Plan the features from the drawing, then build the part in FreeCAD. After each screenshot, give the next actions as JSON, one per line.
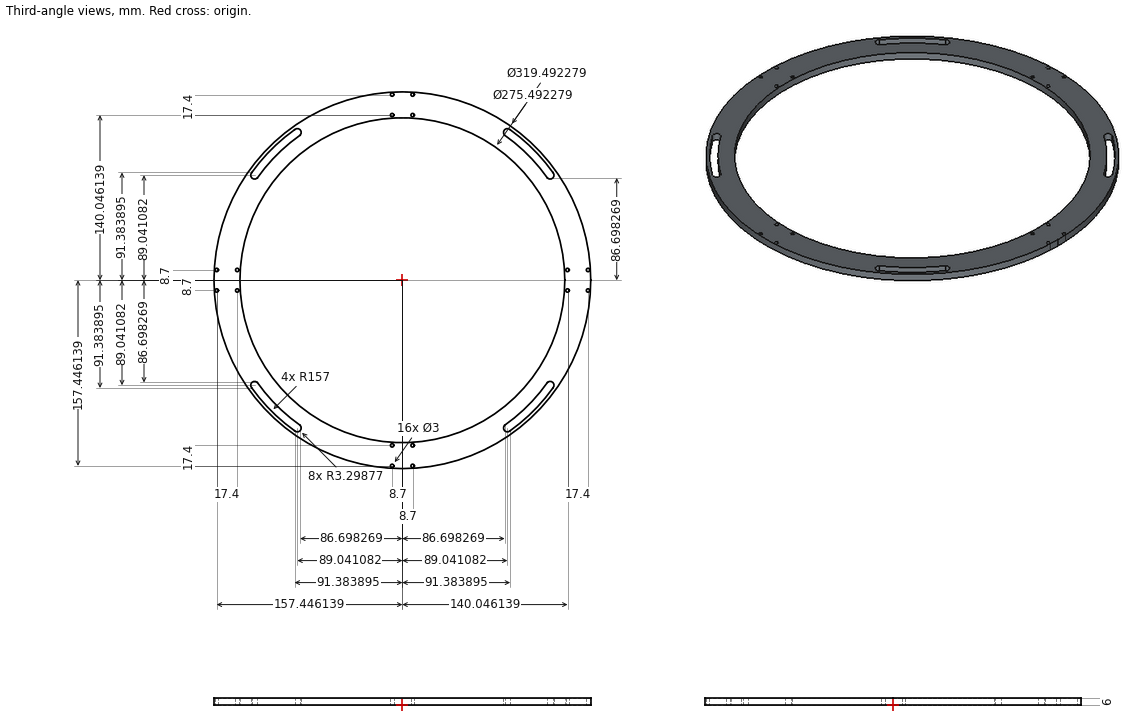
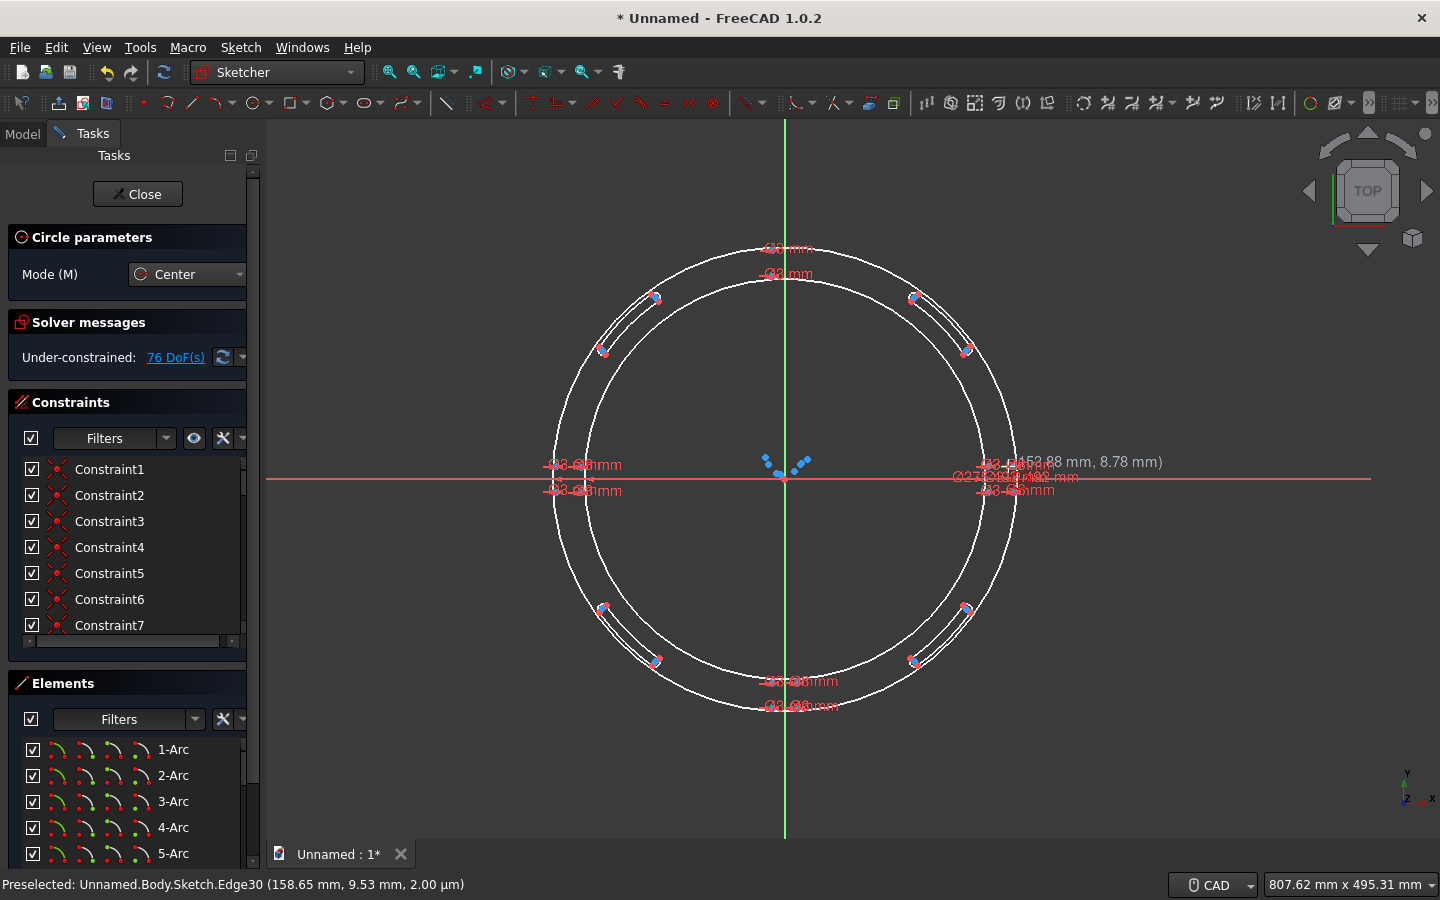
{"action": "scroll", "coordinate": [798, 276], "scroll_direction": "up", "scroll_amount": 12}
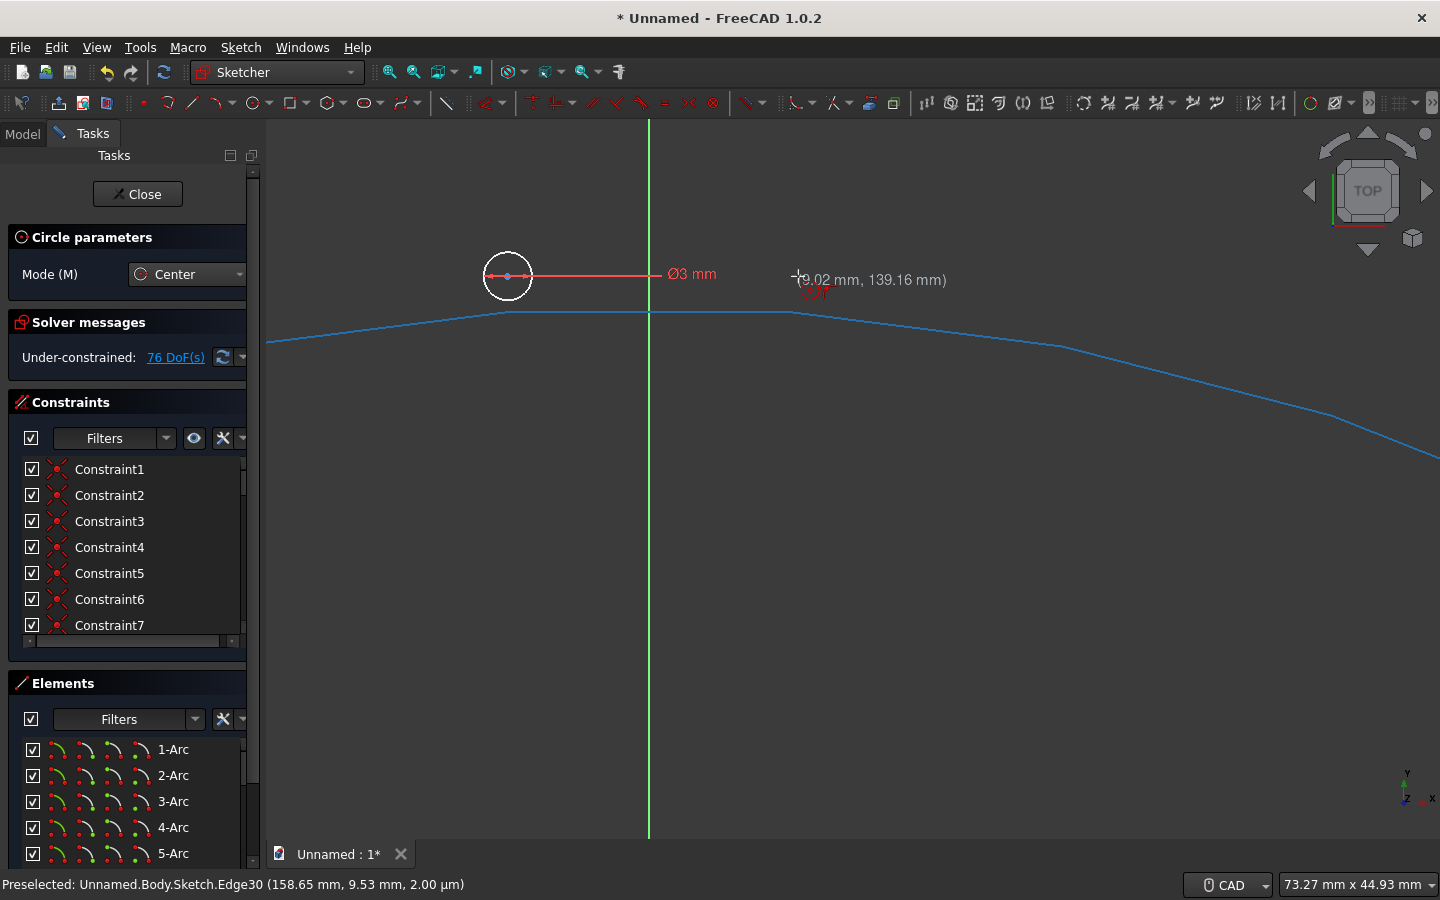
{"action": "left_click", "coordinate": [788, 271]}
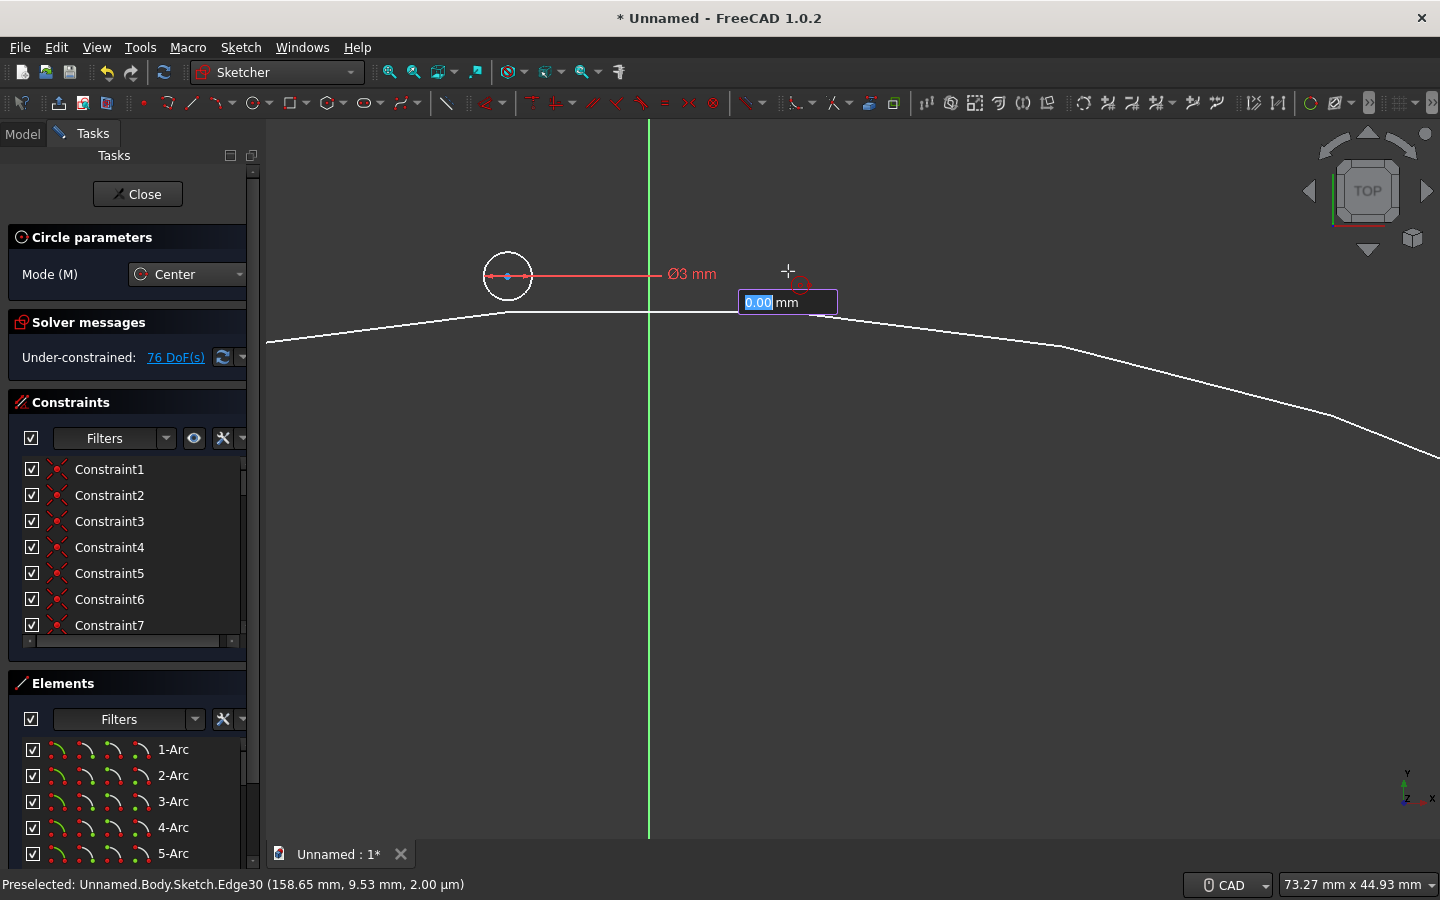
{"action": "scroll", "coordinate": [798, 276], "scroll_direction": "down", "scroll_amount": 12}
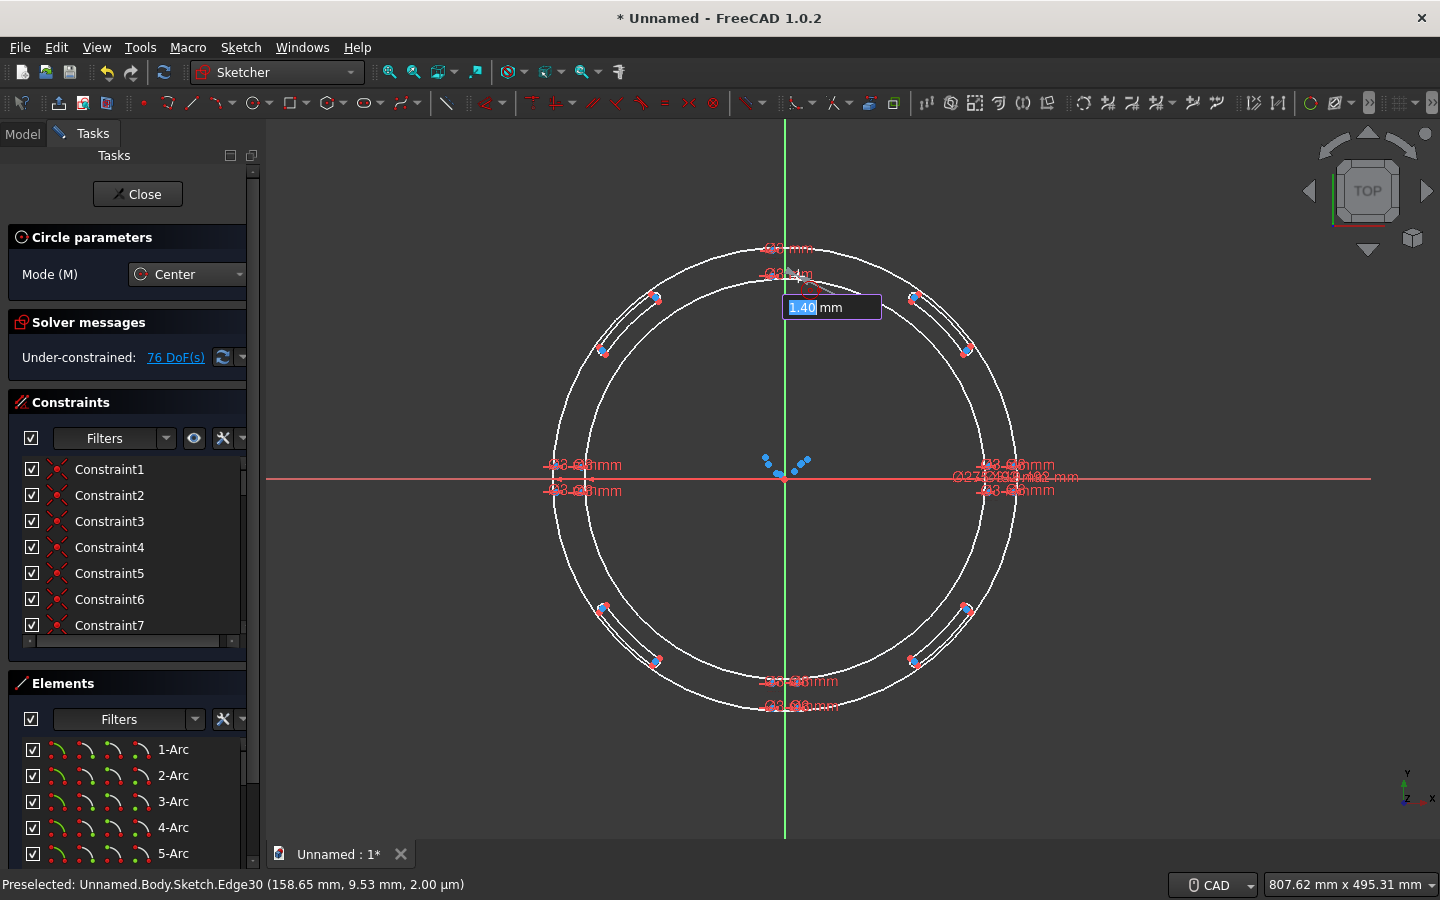
{"action": "scroll", "coordinate": [799, 274], "scroll_direction": "up", "scroll_amount": 6}
{"action": "mouse_move", "coordinate": [798, 274]}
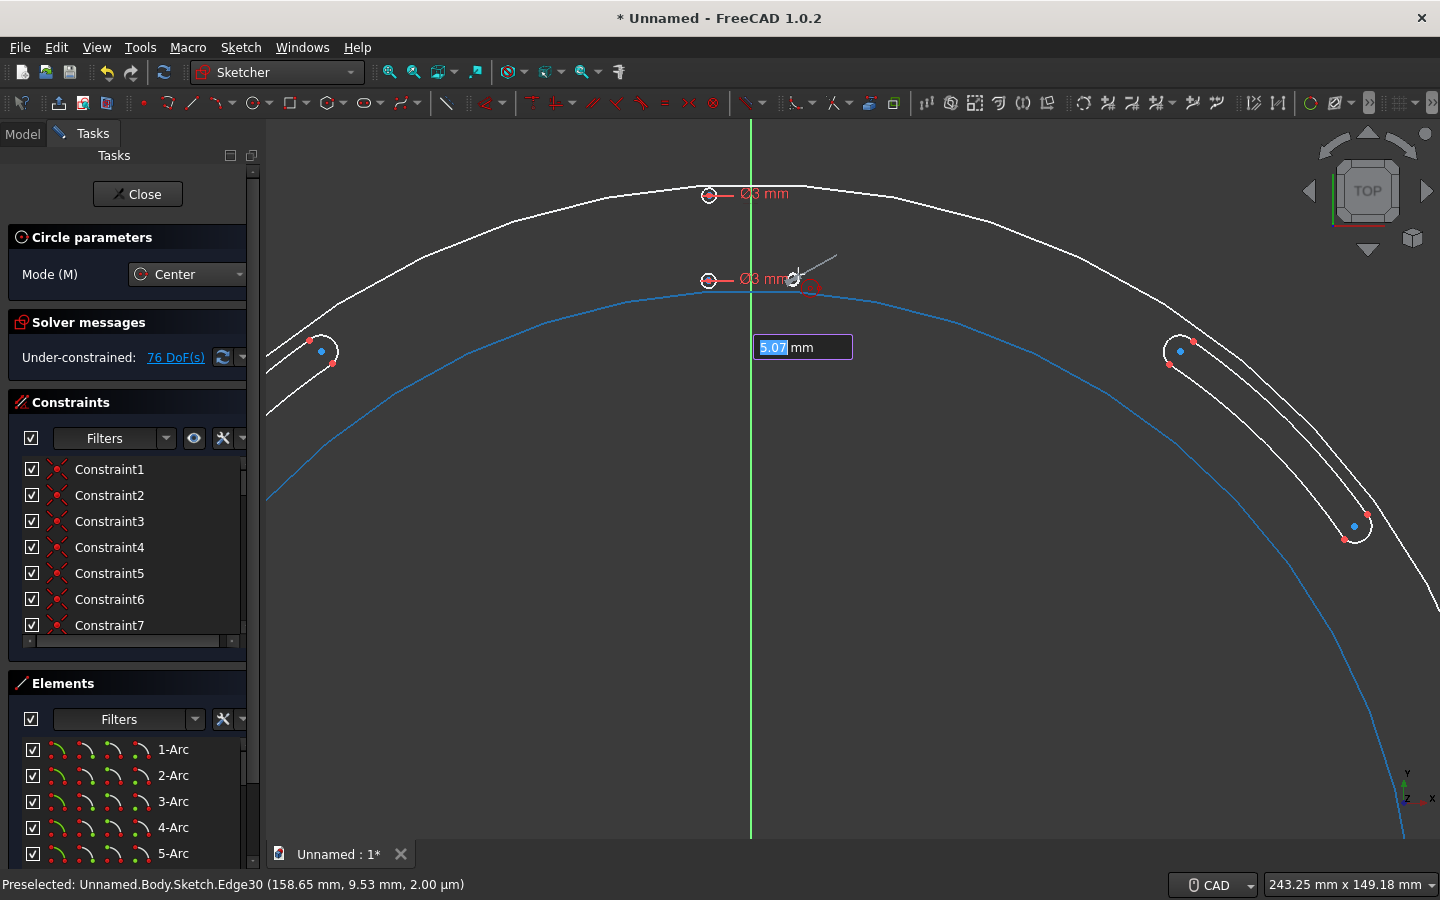
{"action": "type", "text": "3"}
{"action": "key", "text": "Return"}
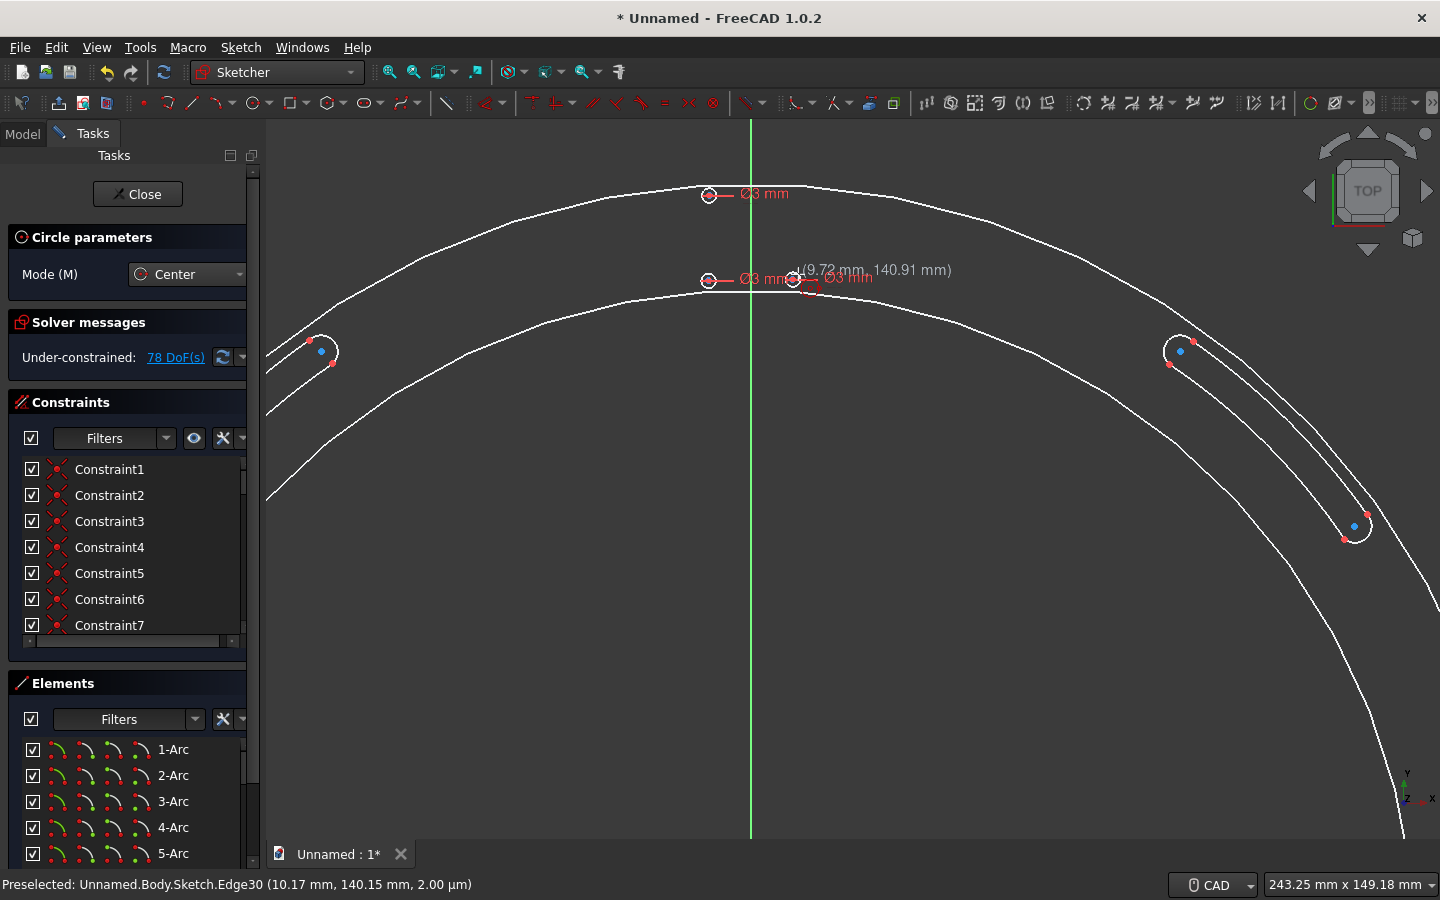
{"action": "scroll", "coordinate": [793, 195], "scroll_direction": "up", "scroll_amount": 6}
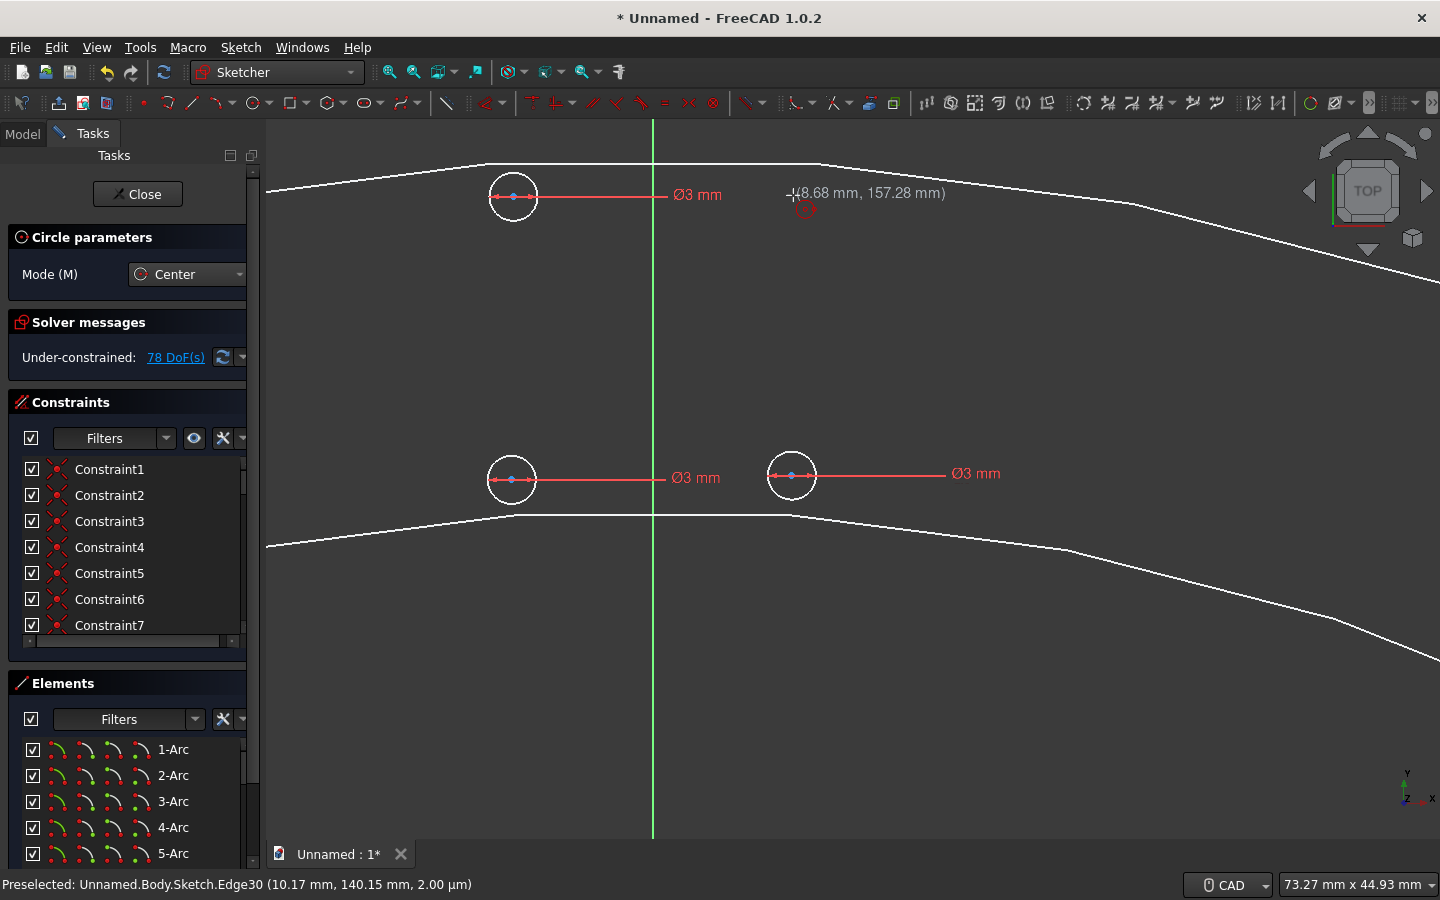
{"action": "left_click", "coordinate": [792, 195]}
{"action": "mouse_move", "coordinate": [809, 178]}